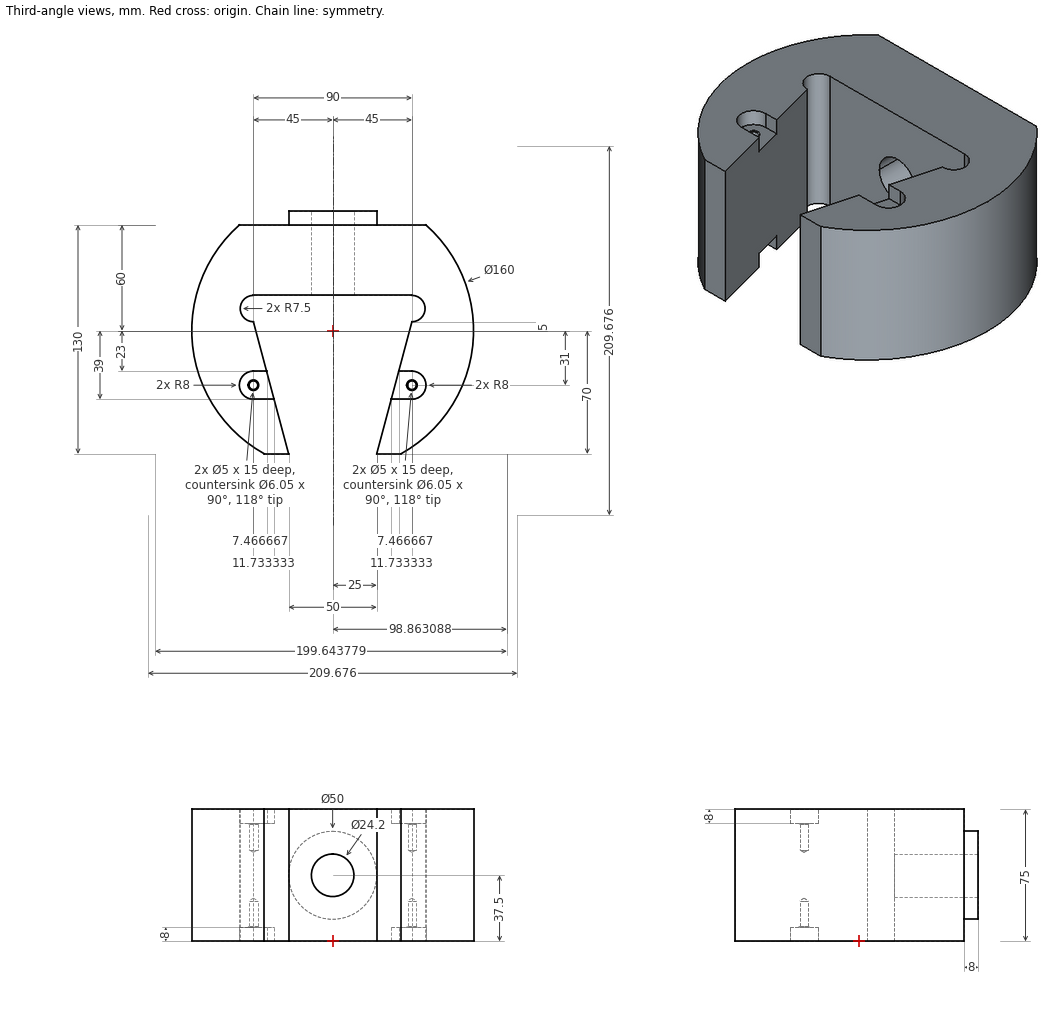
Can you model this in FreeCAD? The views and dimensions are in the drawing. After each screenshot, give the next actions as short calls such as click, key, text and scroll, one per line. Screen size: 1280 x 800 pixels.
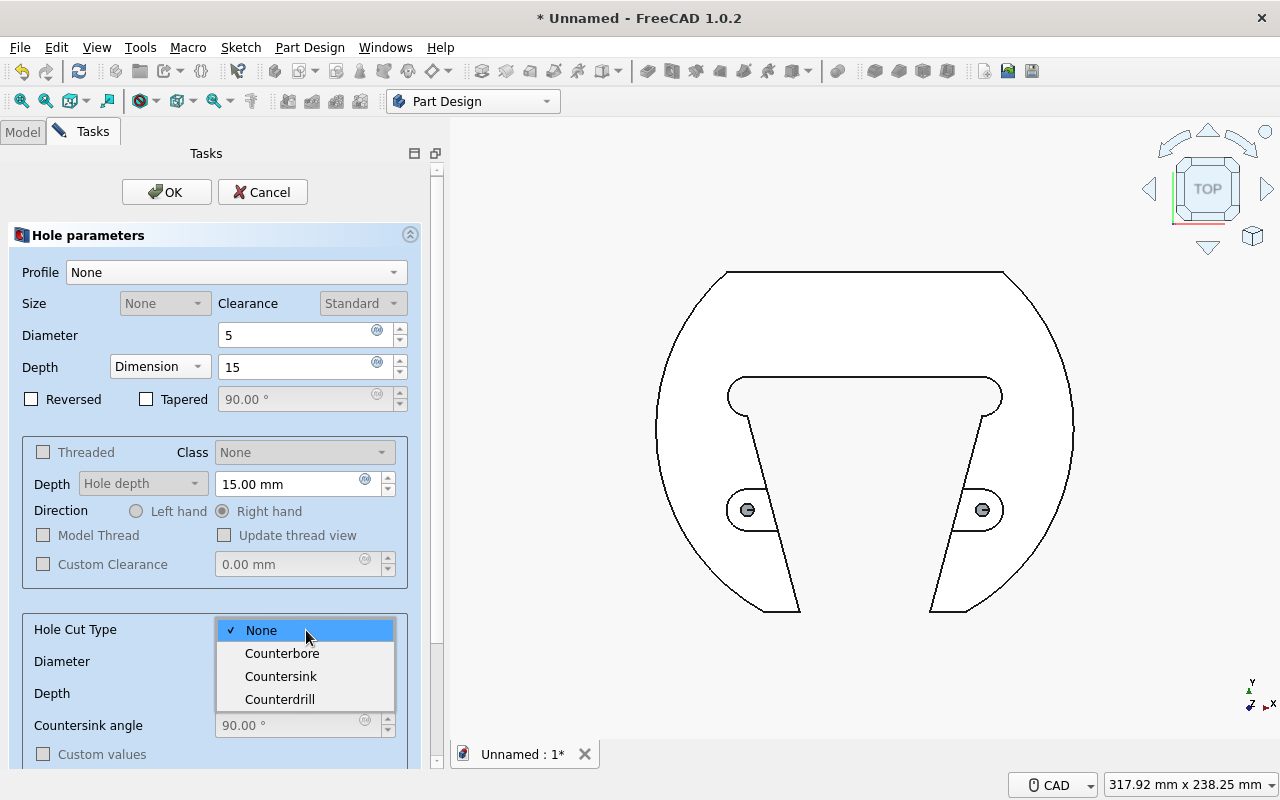
click(304, 676)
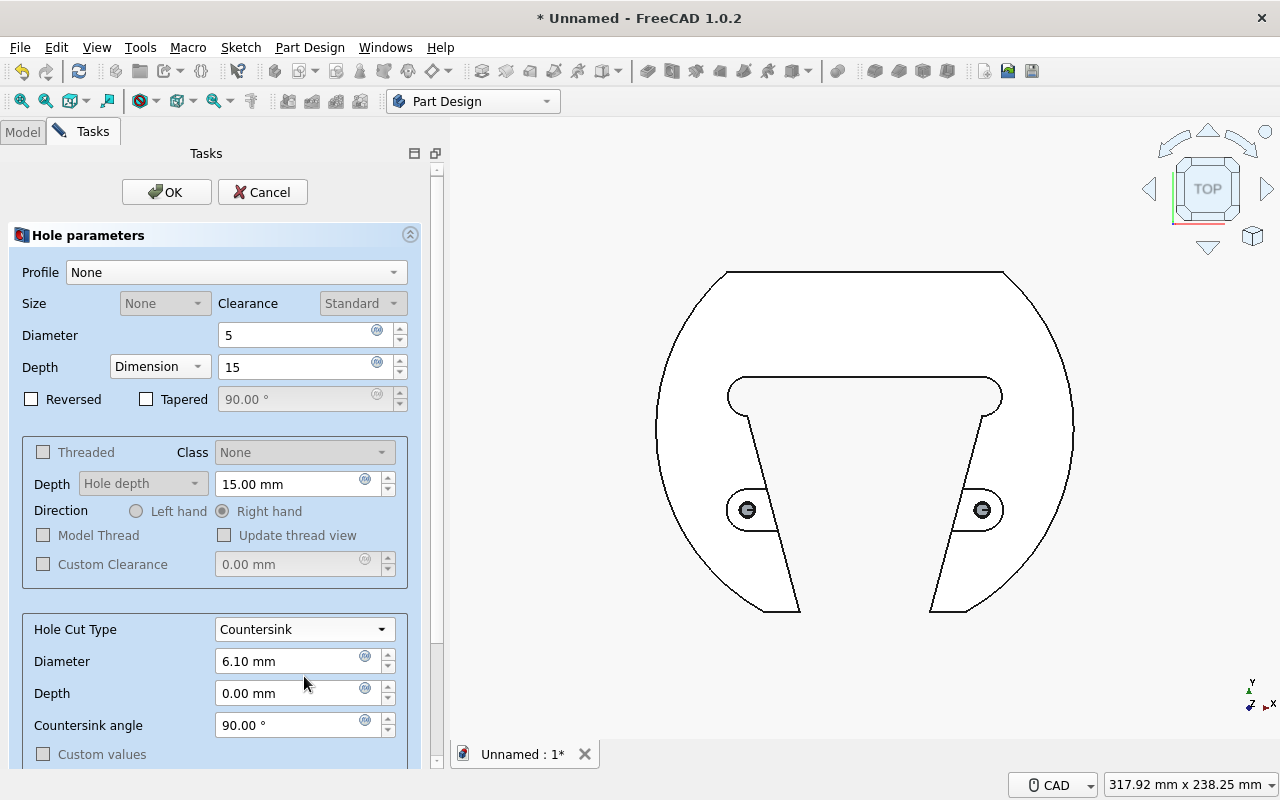
triple_click(298, 661)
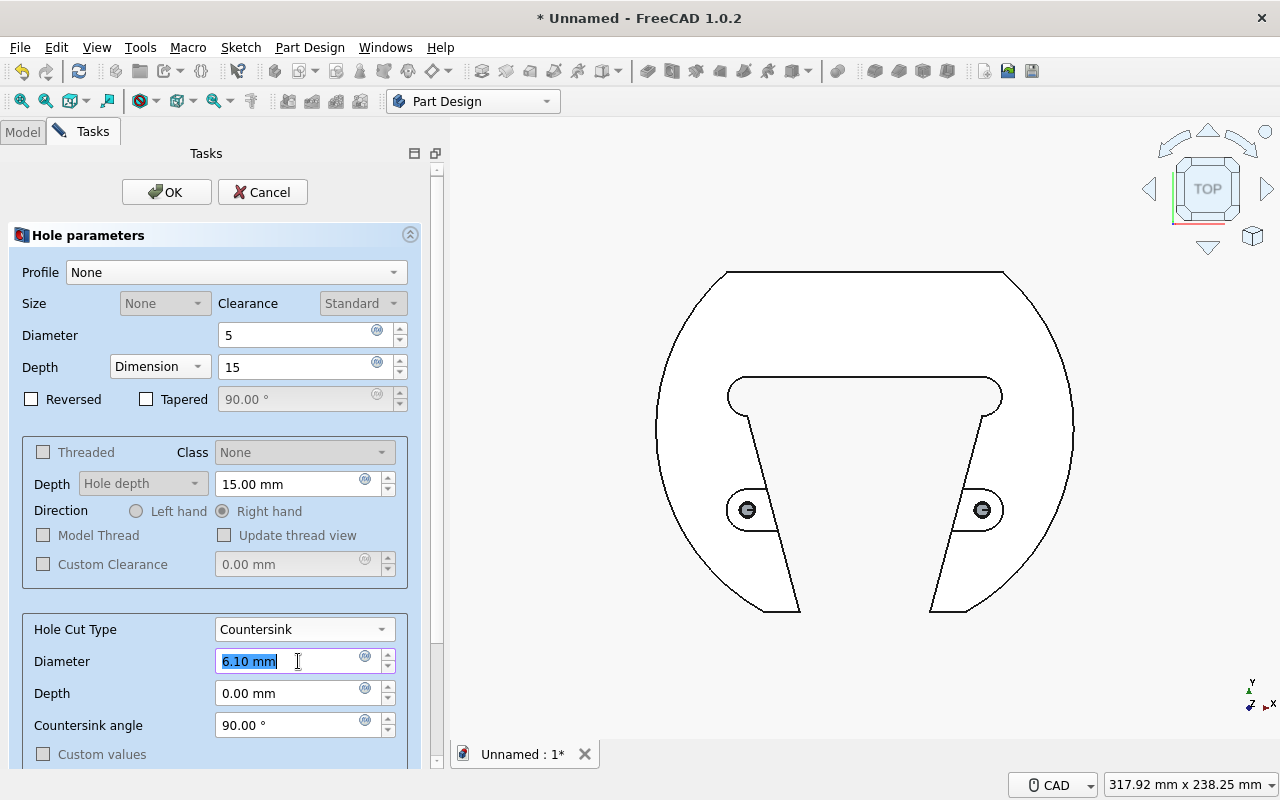
text(6.05)
key(Tab)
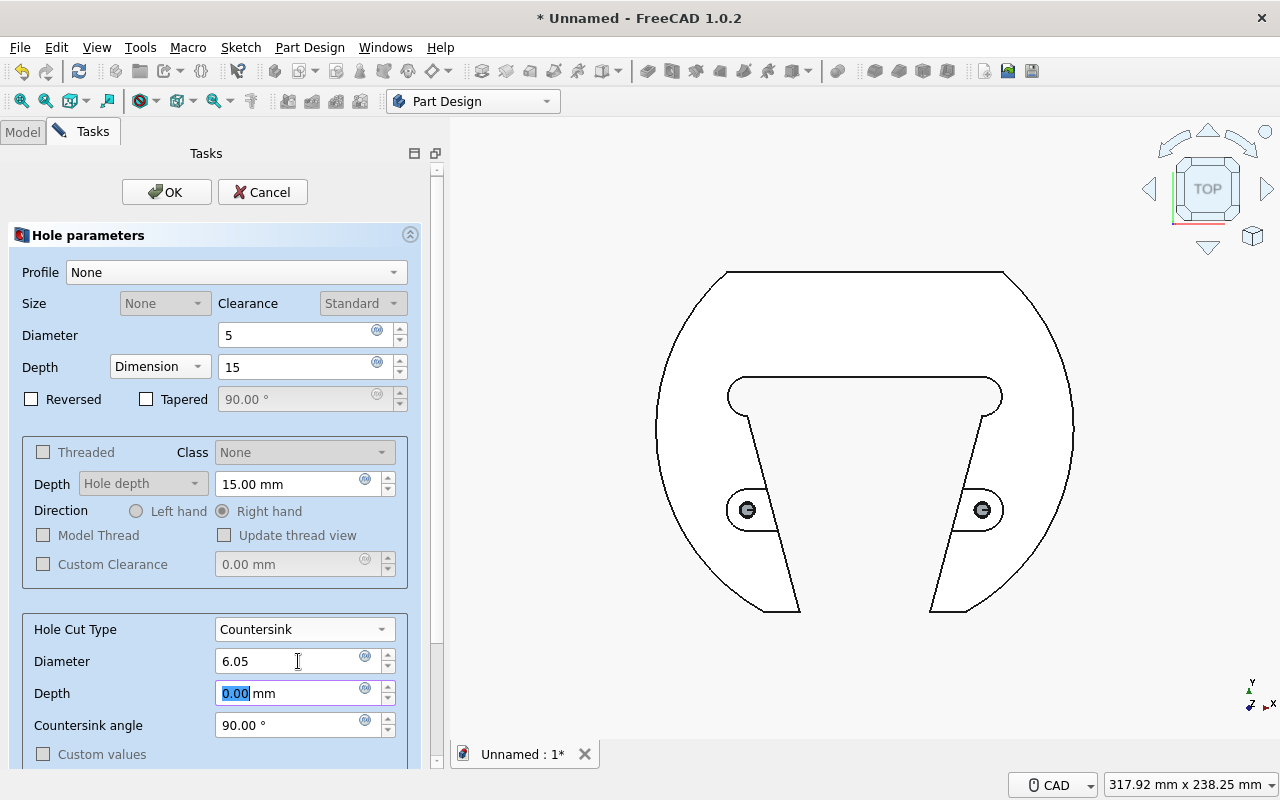
click(167, 192)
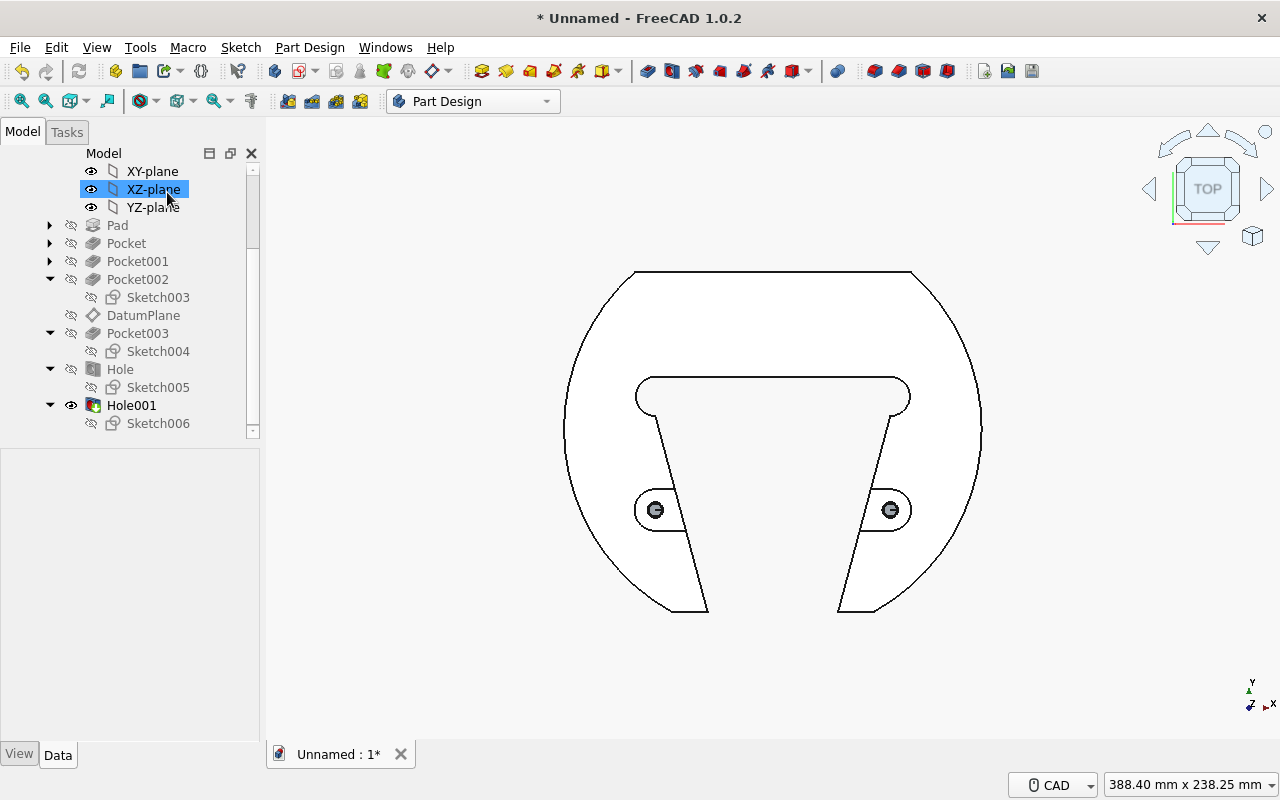
key(4)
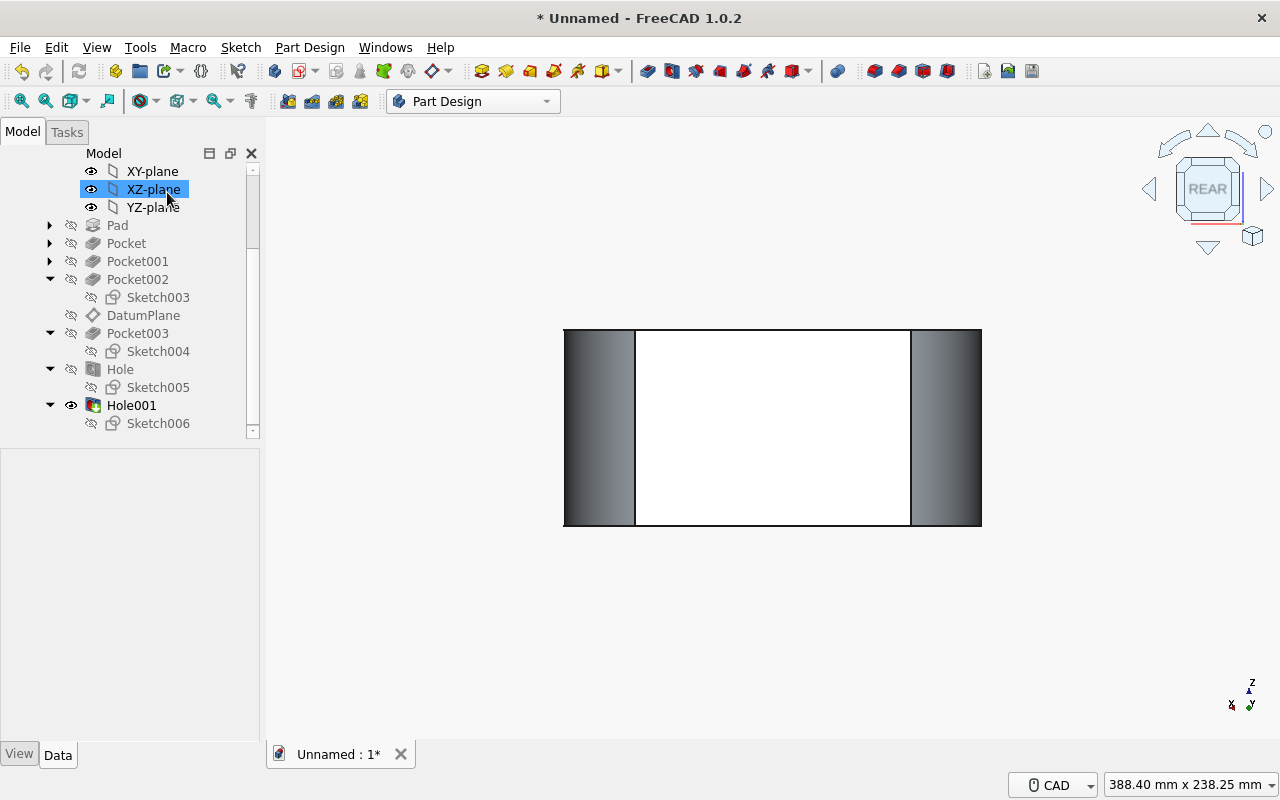
key(v)
key(f)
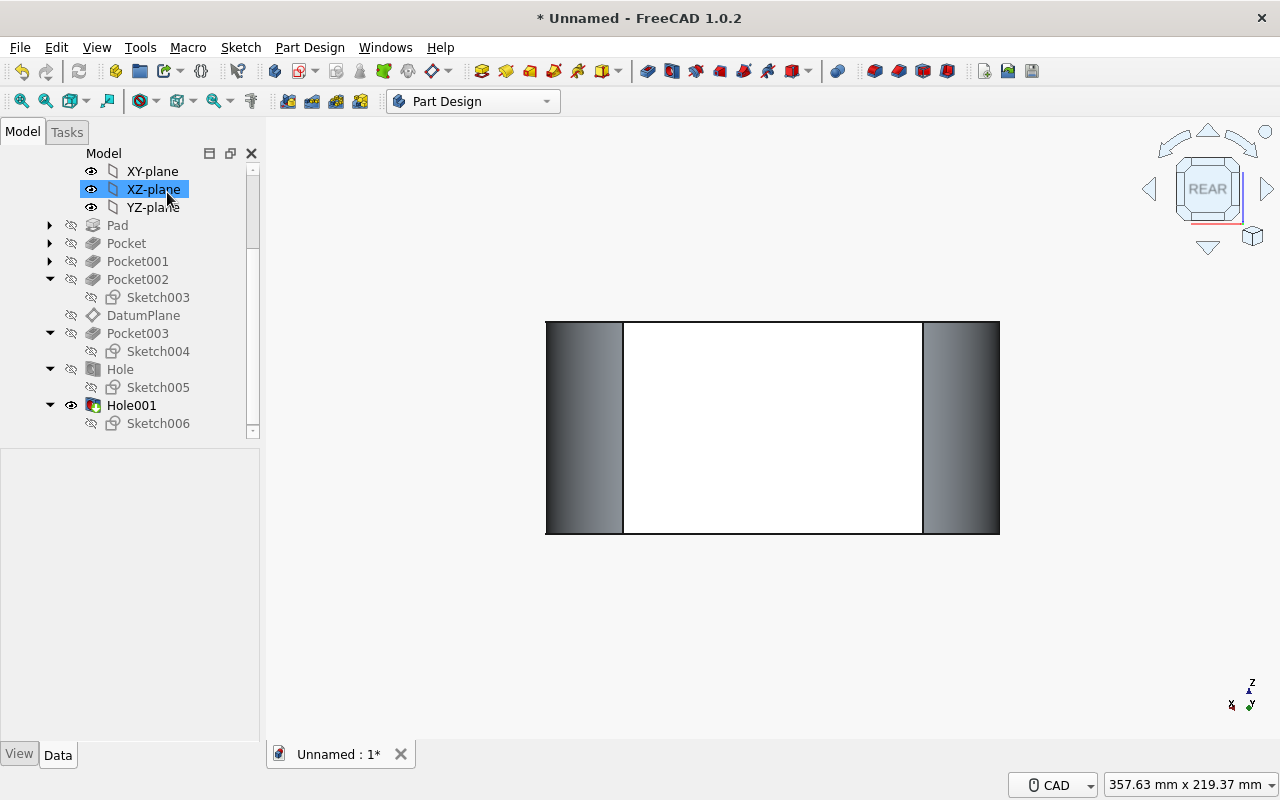
click(730, 427)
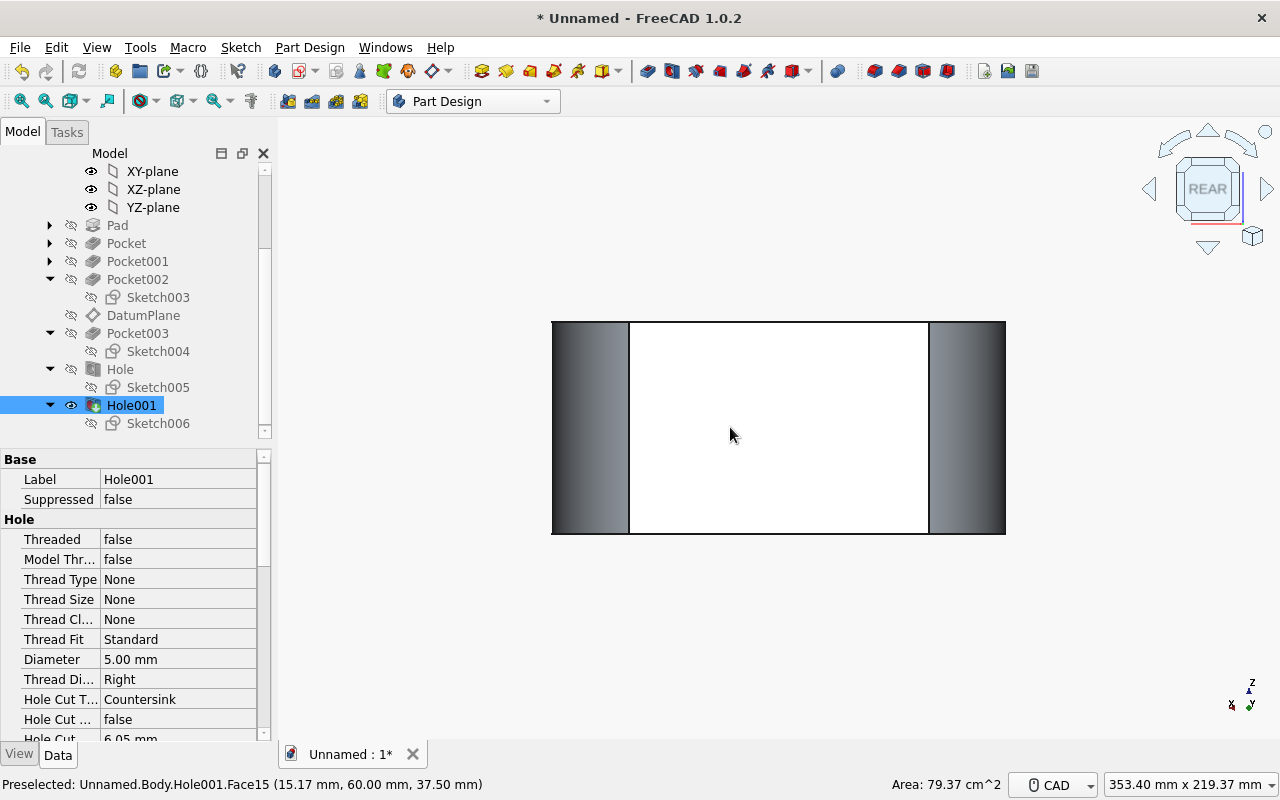
click(300, 72)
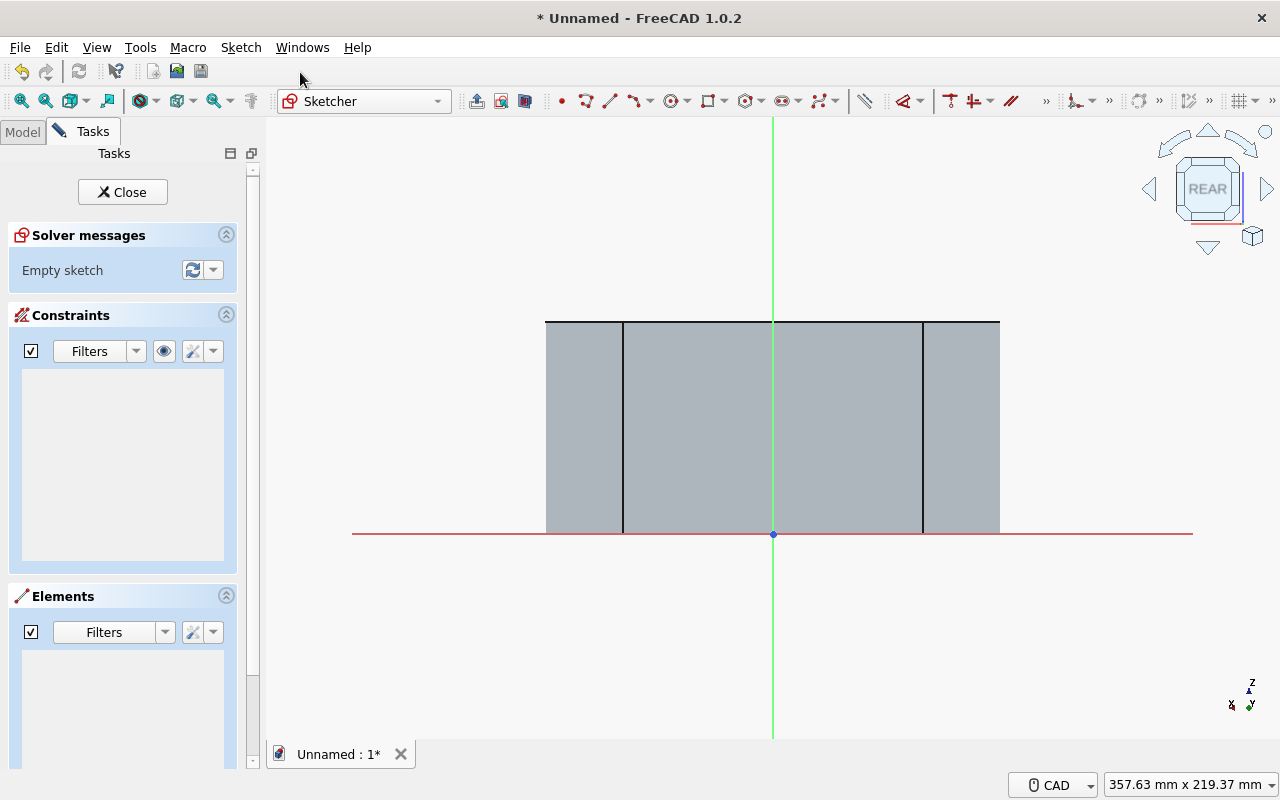
scroll(813, 485, up, 5)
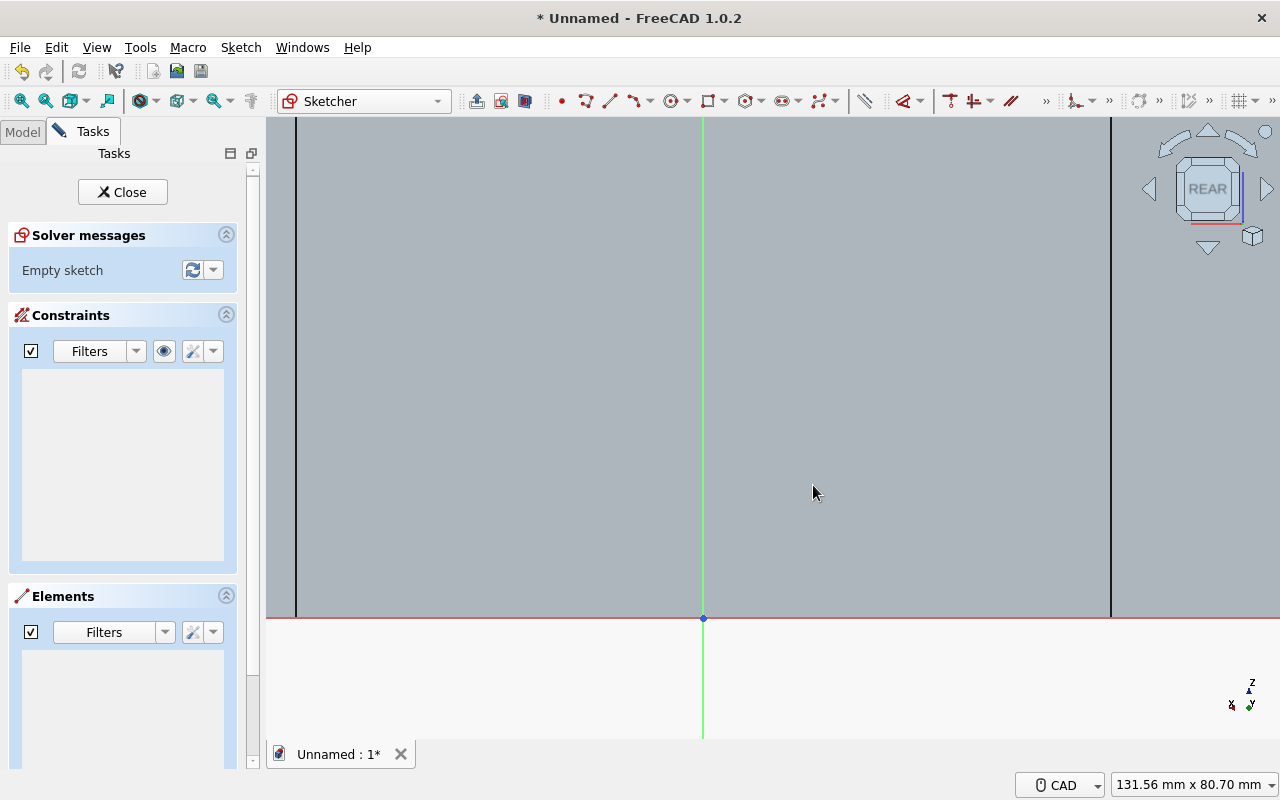
key(g)
key(c)